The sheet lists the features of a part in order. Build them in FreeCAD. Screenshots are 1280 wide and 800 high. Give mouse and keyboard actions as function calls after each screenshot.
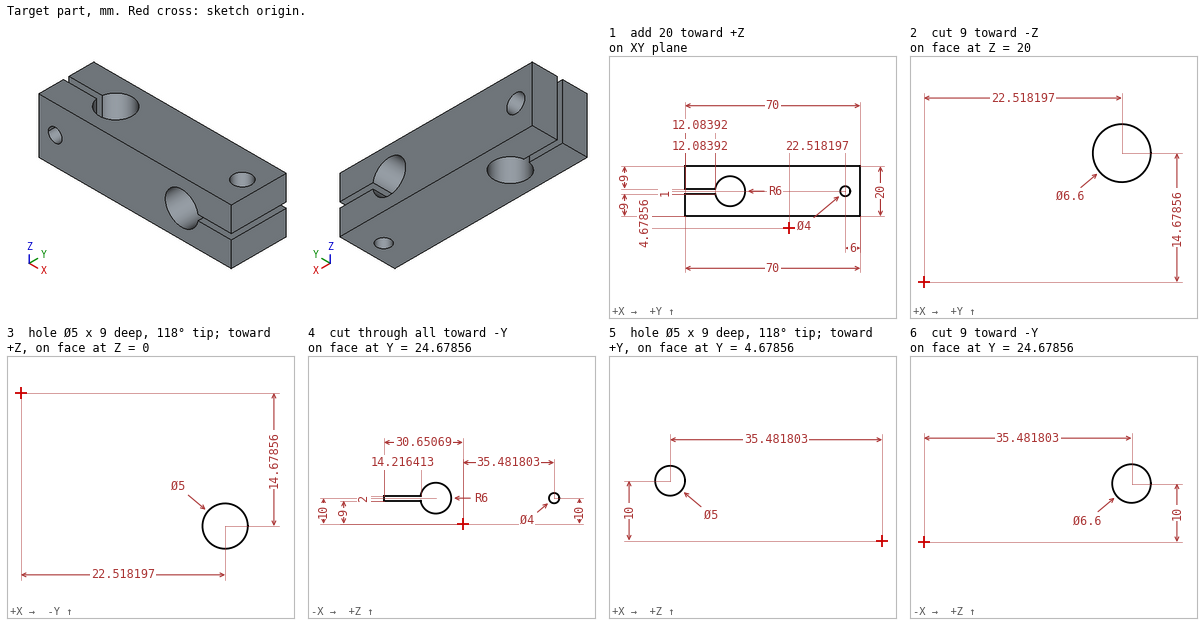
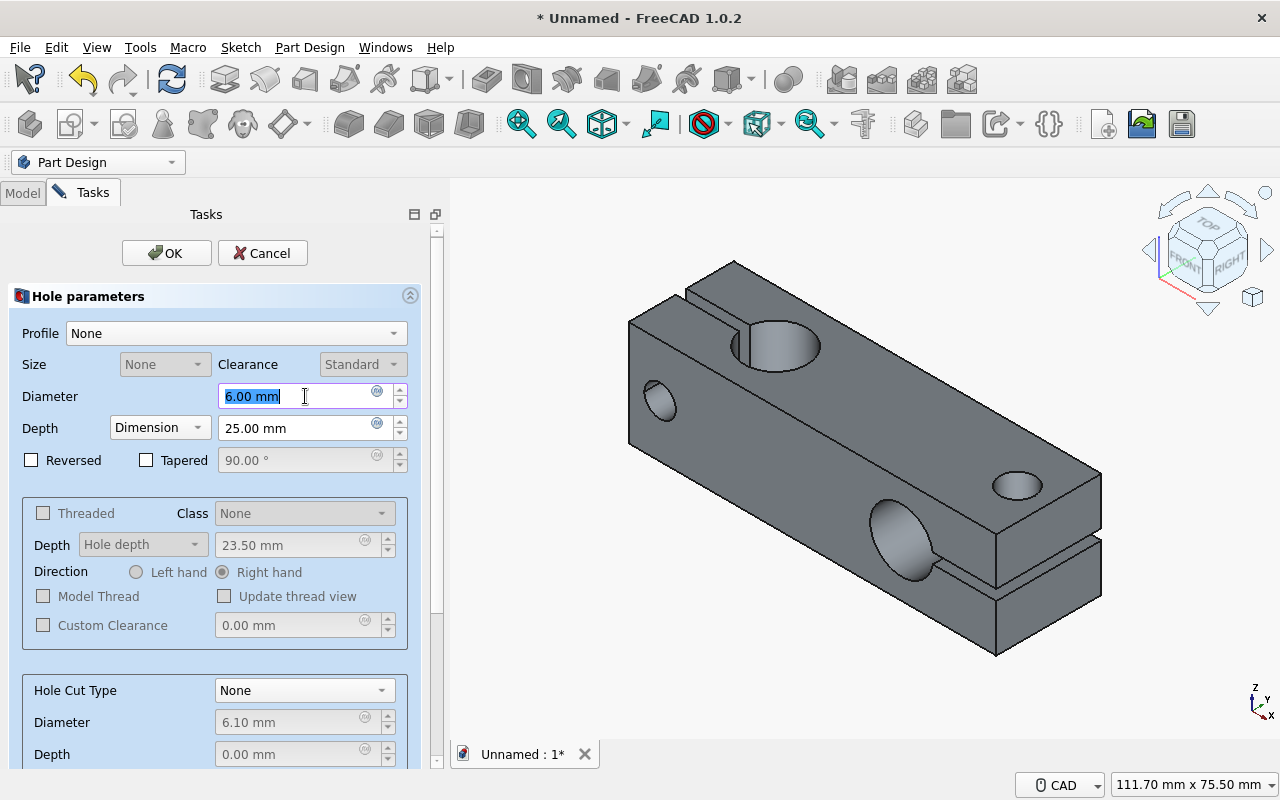
text(5)
key(Tab)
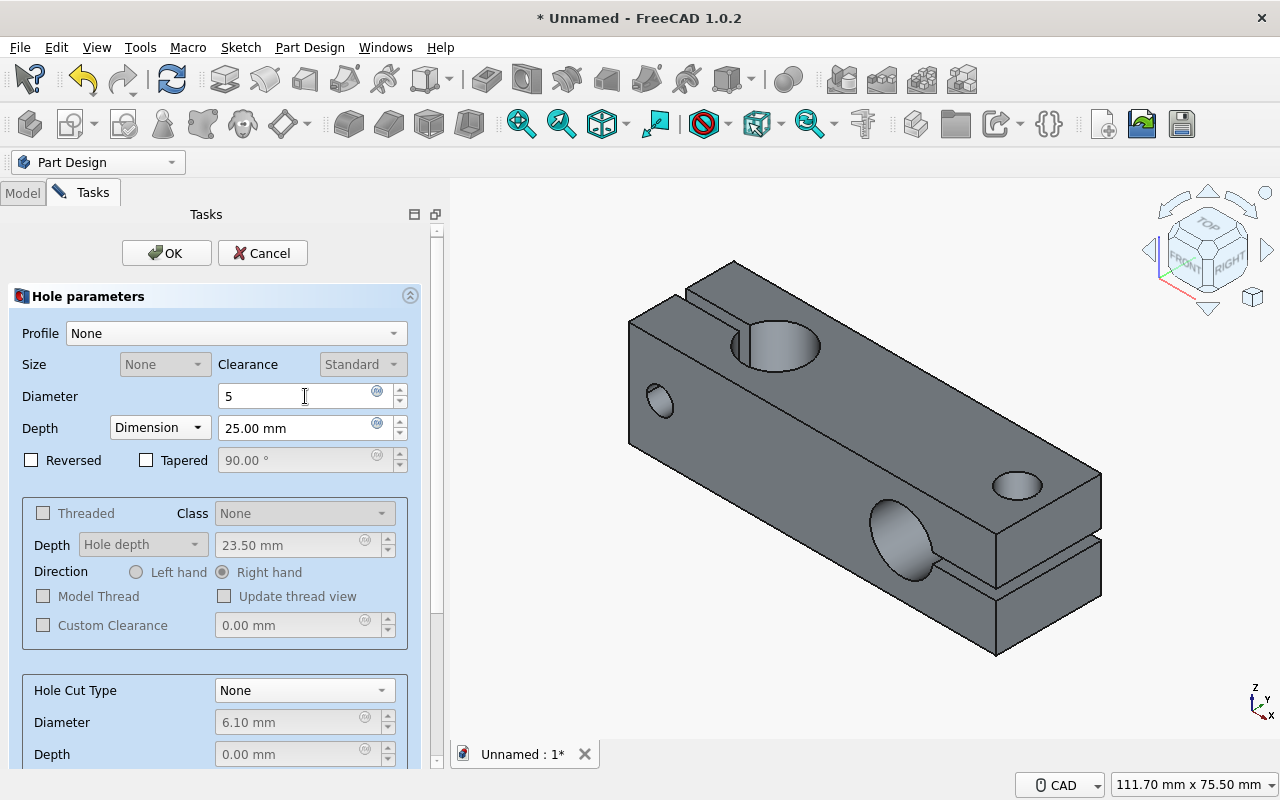
triple_click(305, 428)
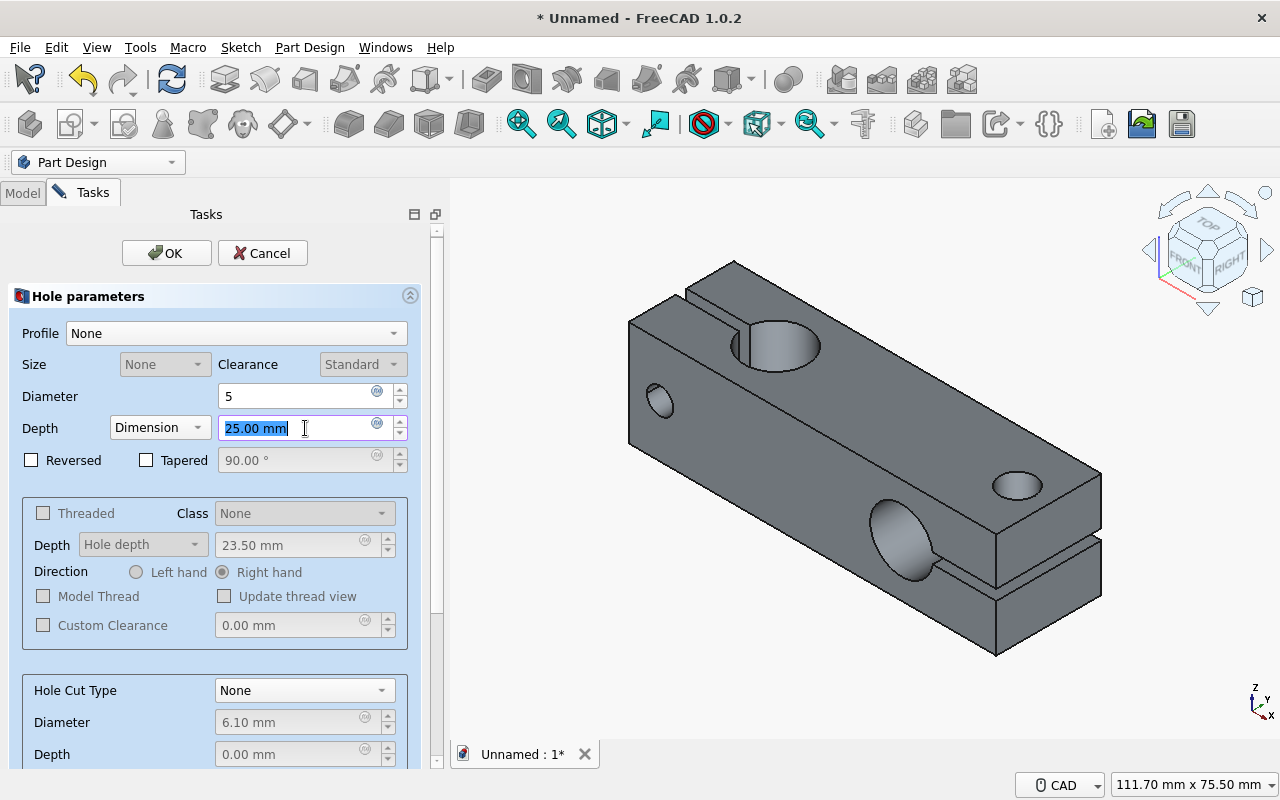
text(9)
key(Tab)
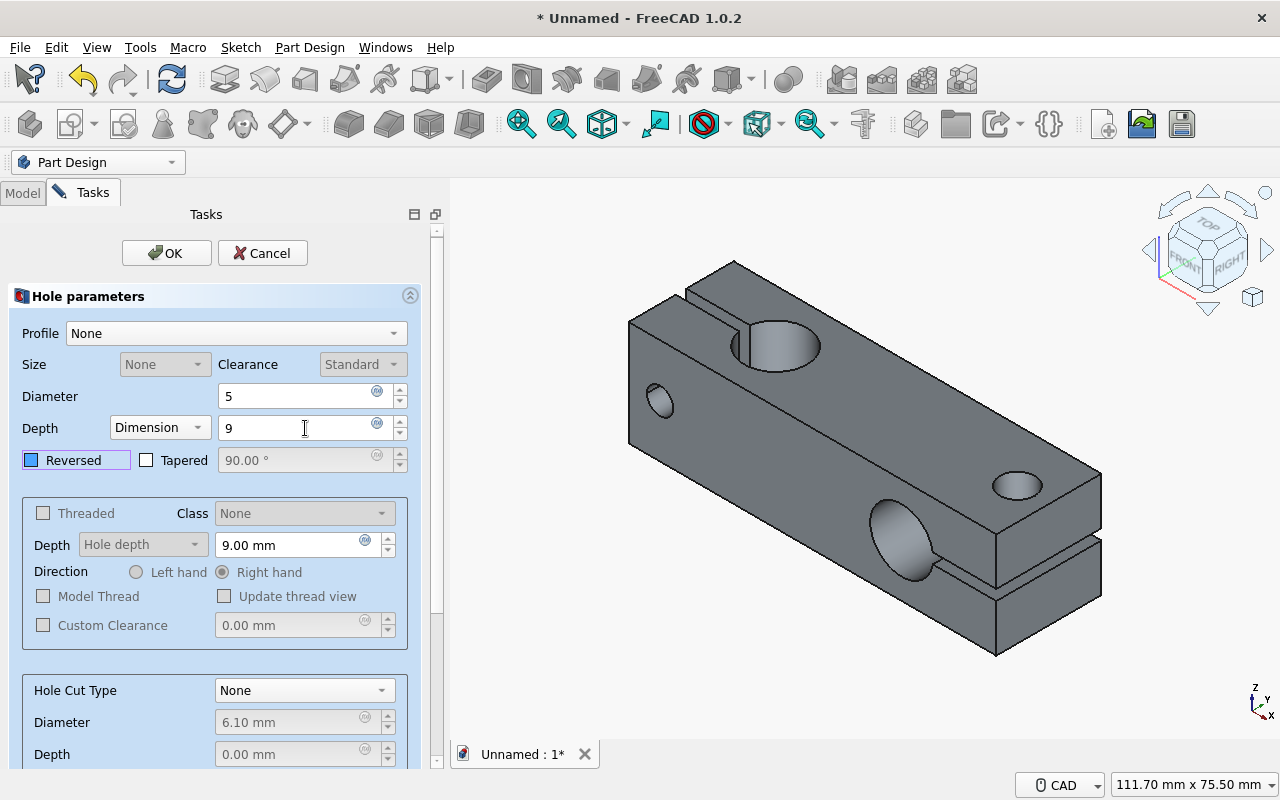
click(167, 253)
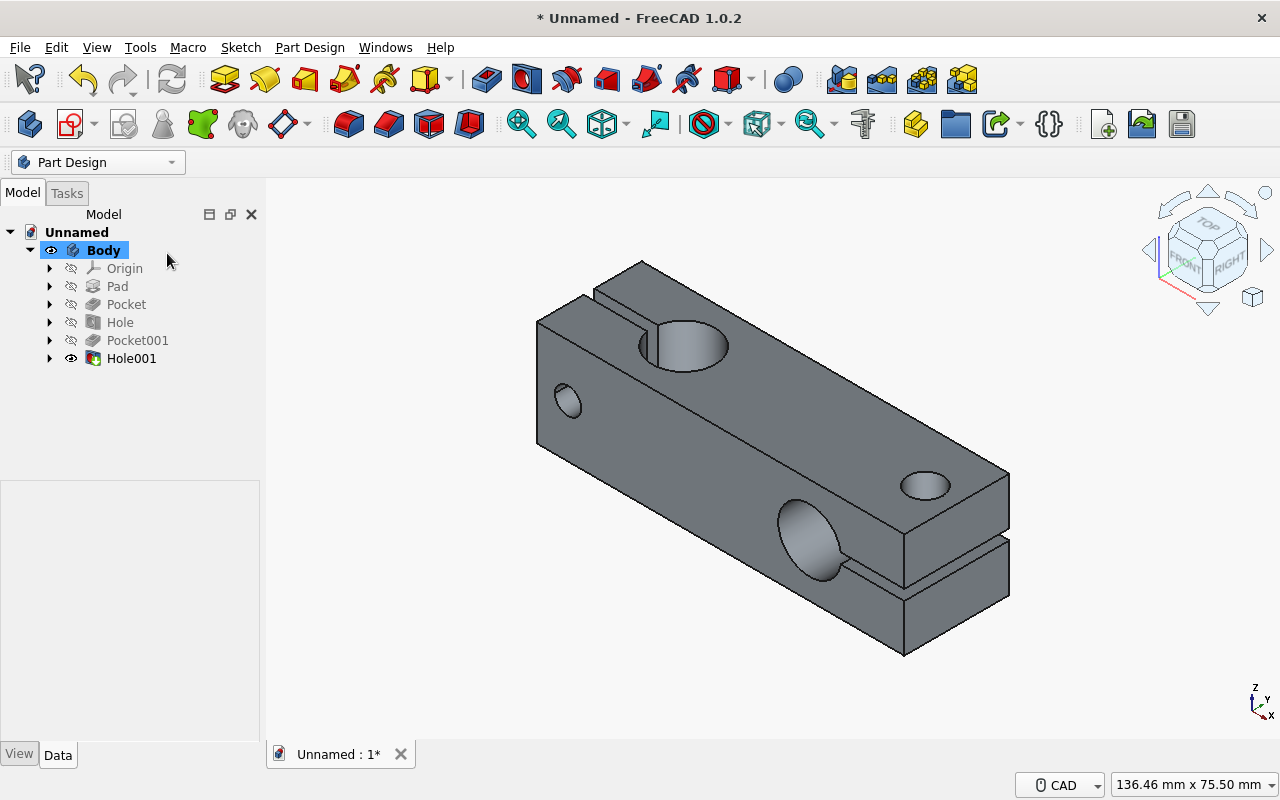
key(4)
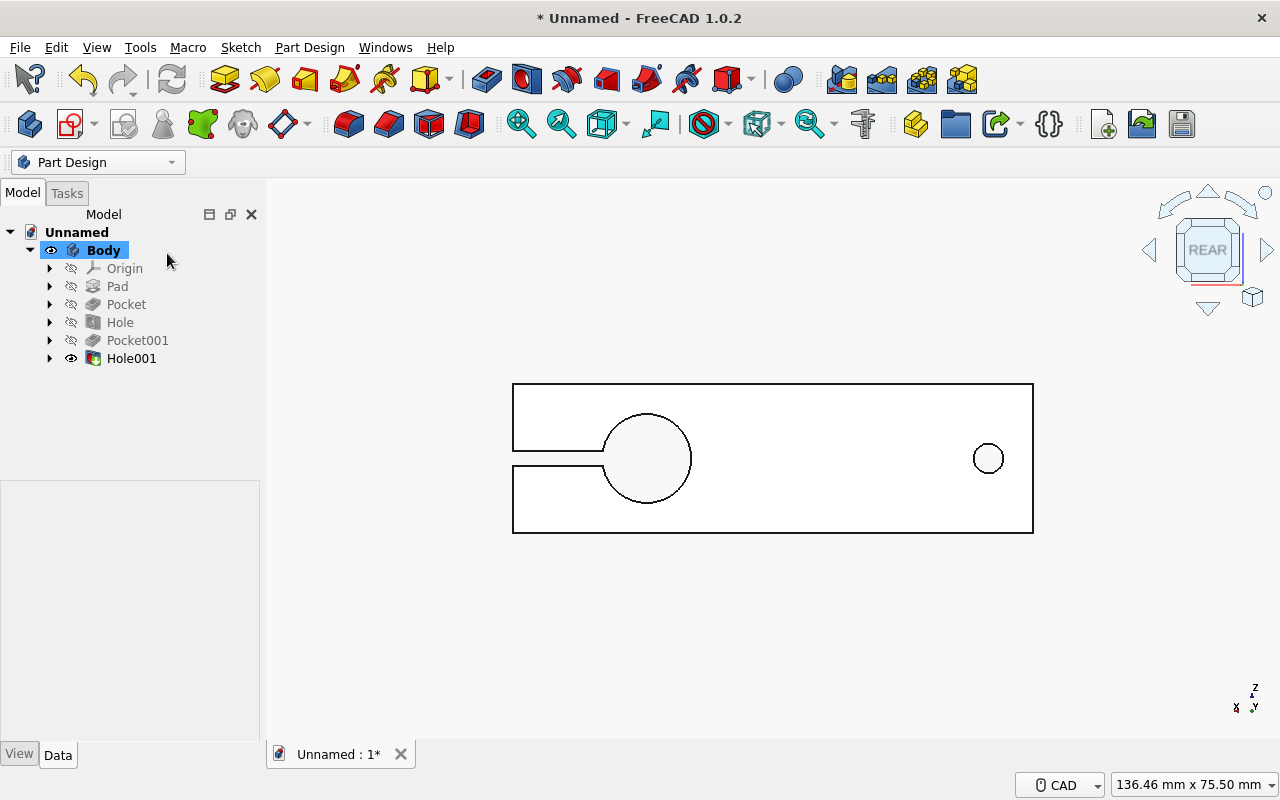
click(773, 458)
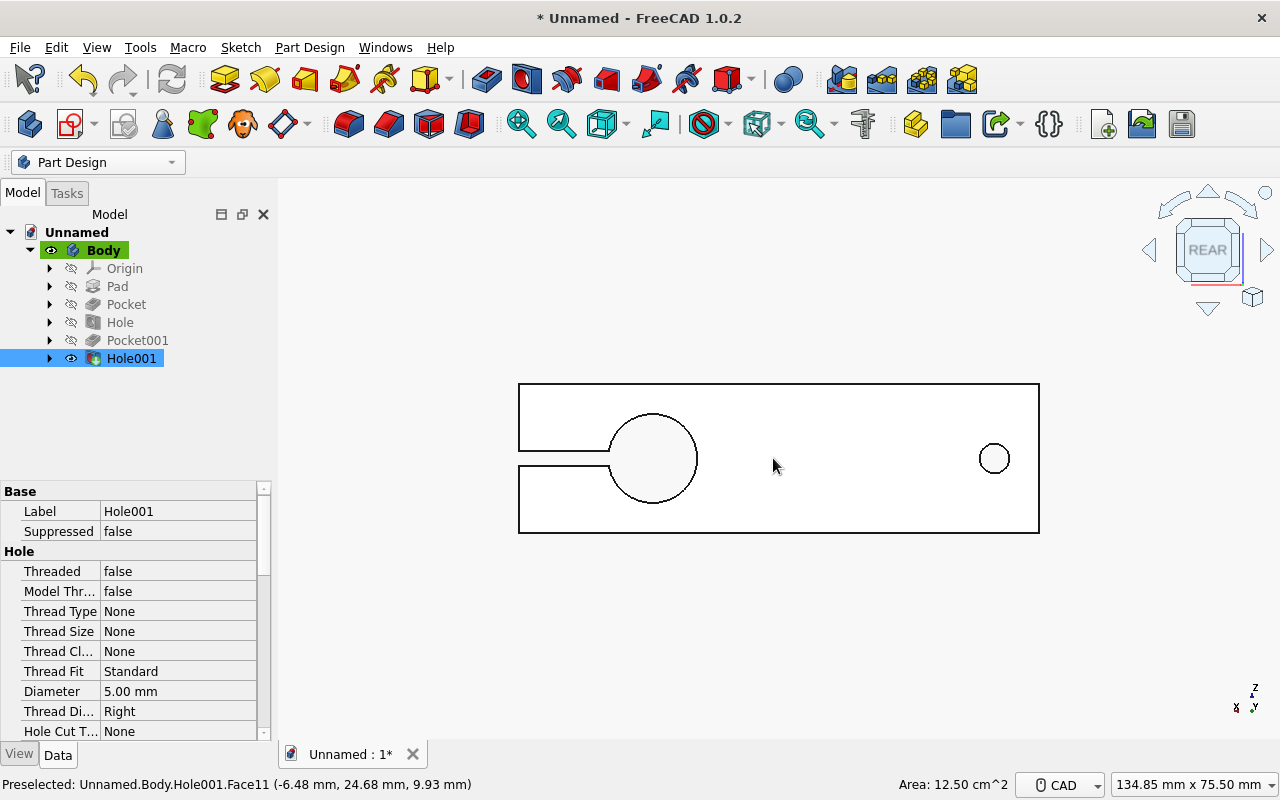
click(70, 124)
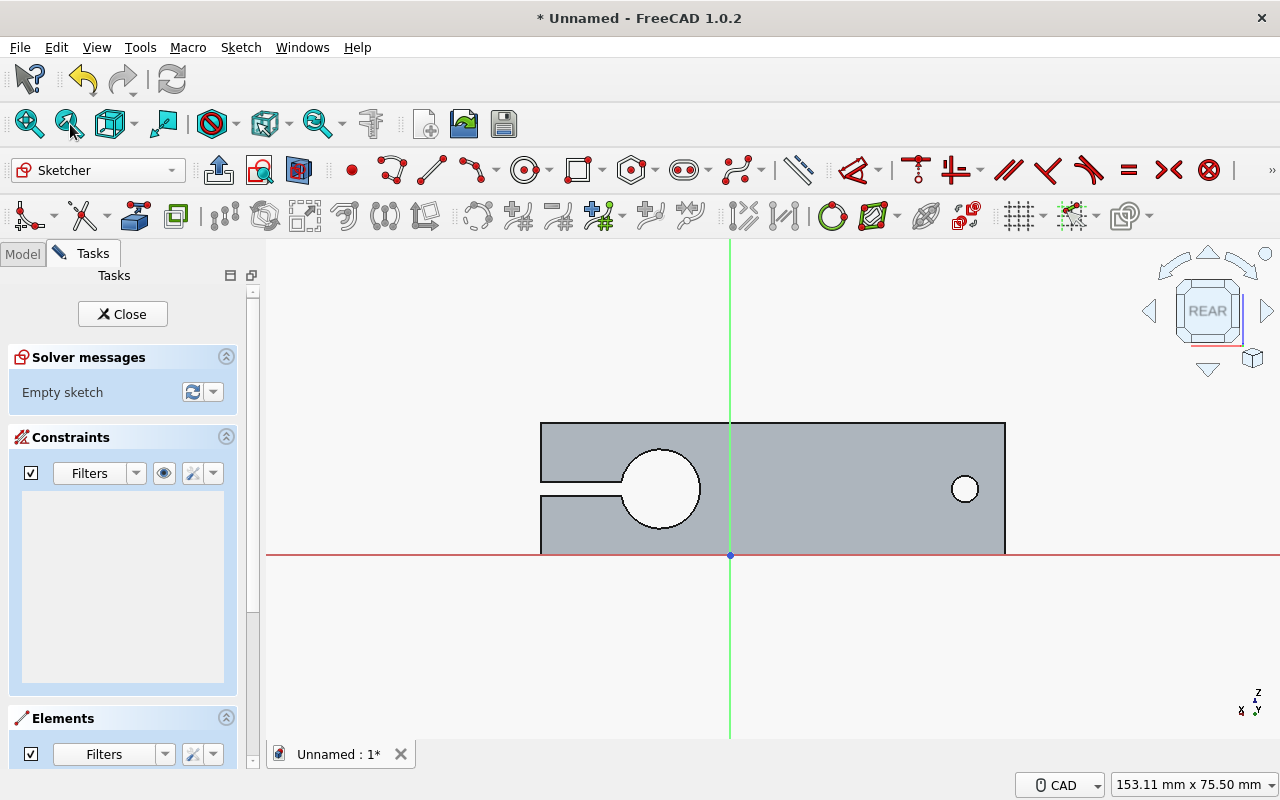
scroll(1006, 489, up, 10)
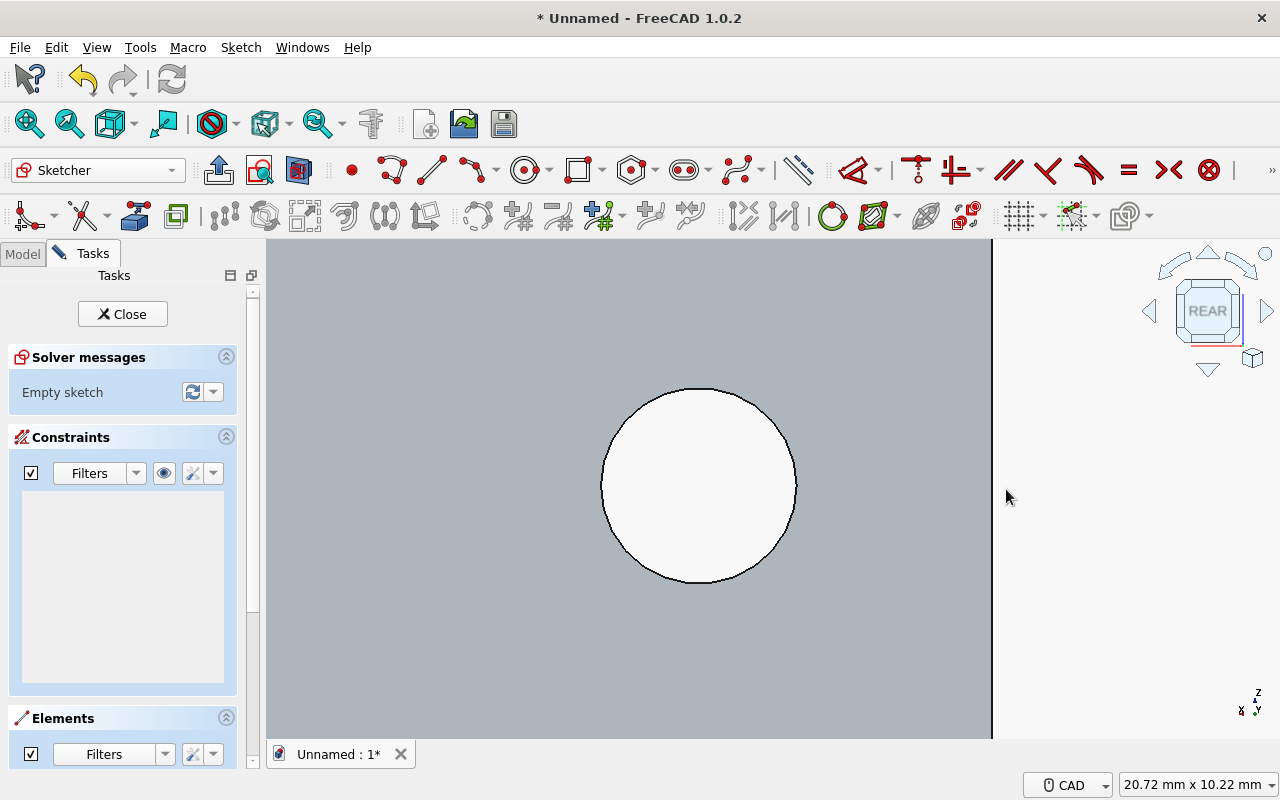
click(526, 170)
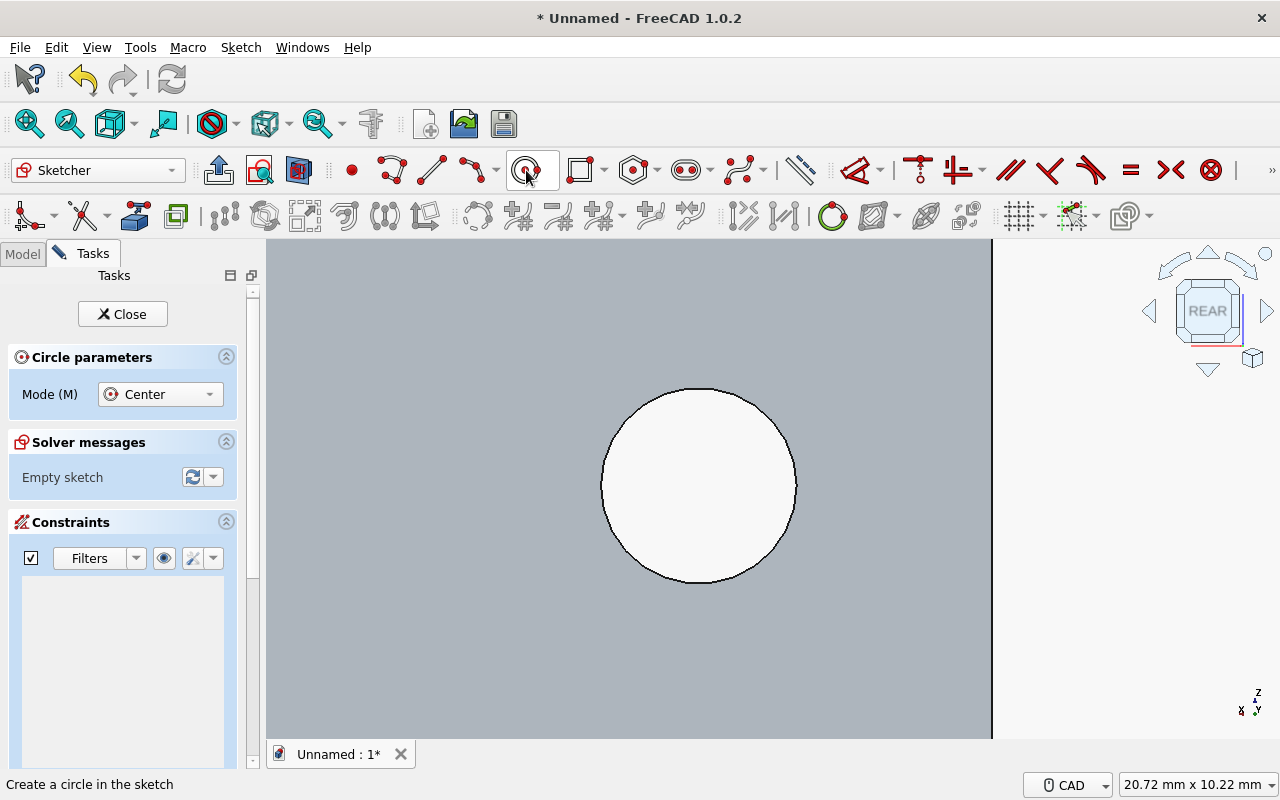
click(699, 486)
click(813, 372)
key(Escape)